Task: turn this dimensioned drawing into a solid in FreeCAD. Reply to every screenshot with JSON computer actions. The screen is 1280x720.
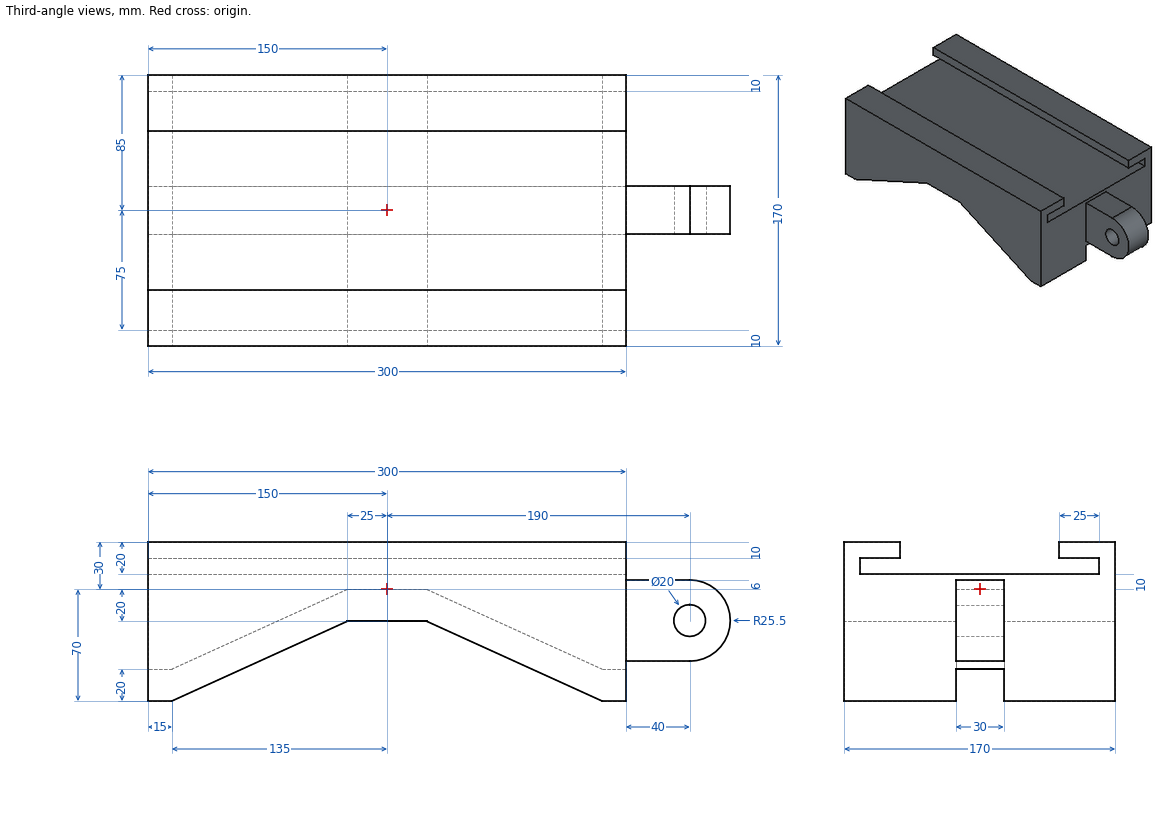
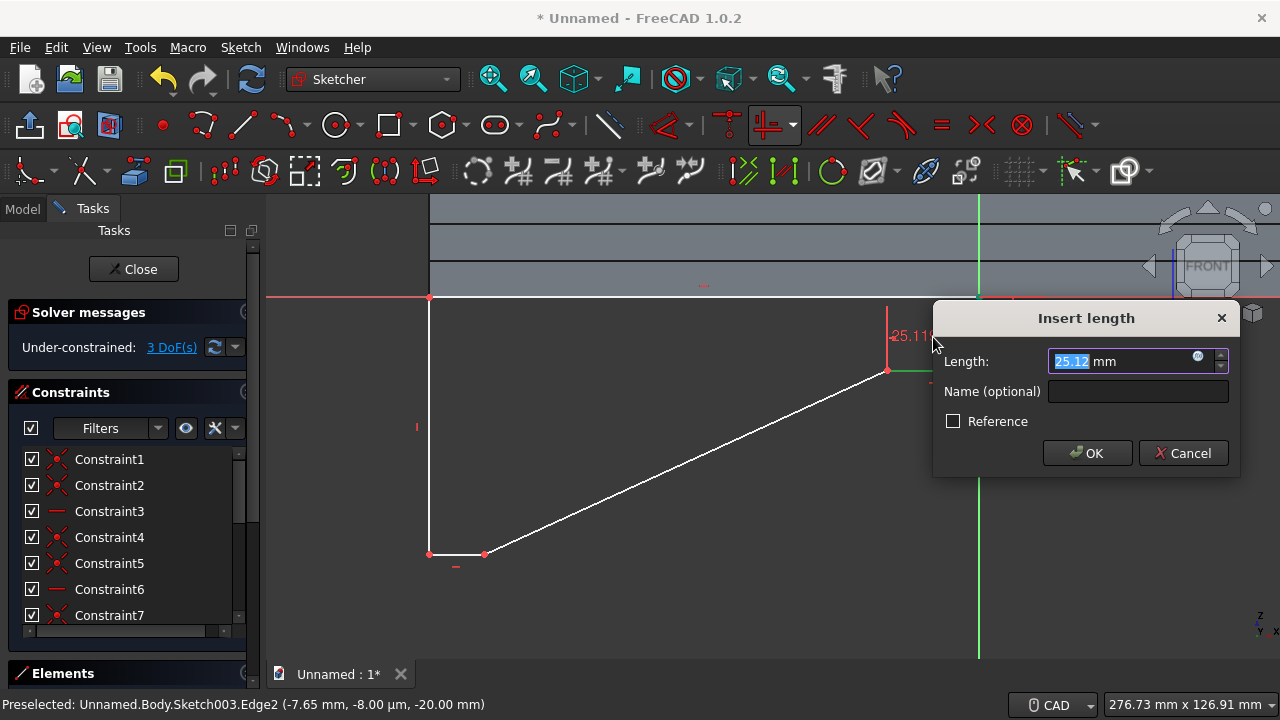
{"action": "type", "text": "25"}
{"action": "key", "text": "Return"}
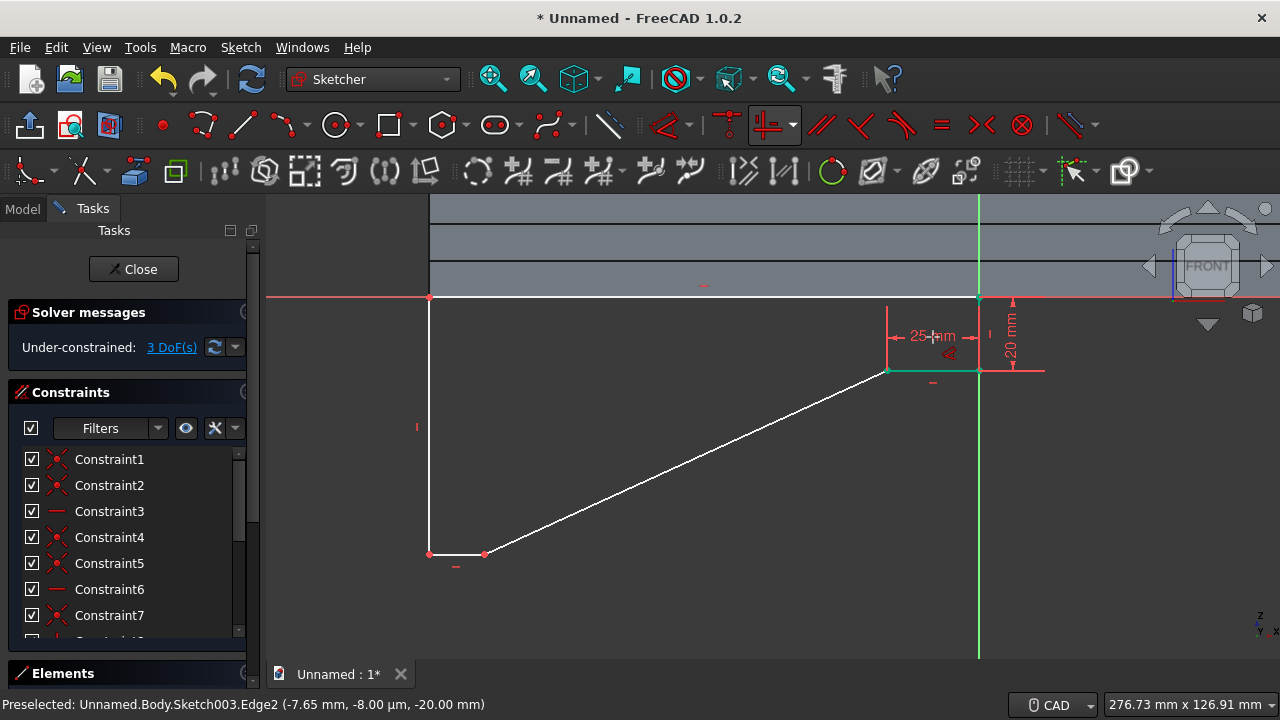
{"action": "left_click", "coordinate": [468, 555]}
{"action": "left_click", "coordinate": [457, 589]}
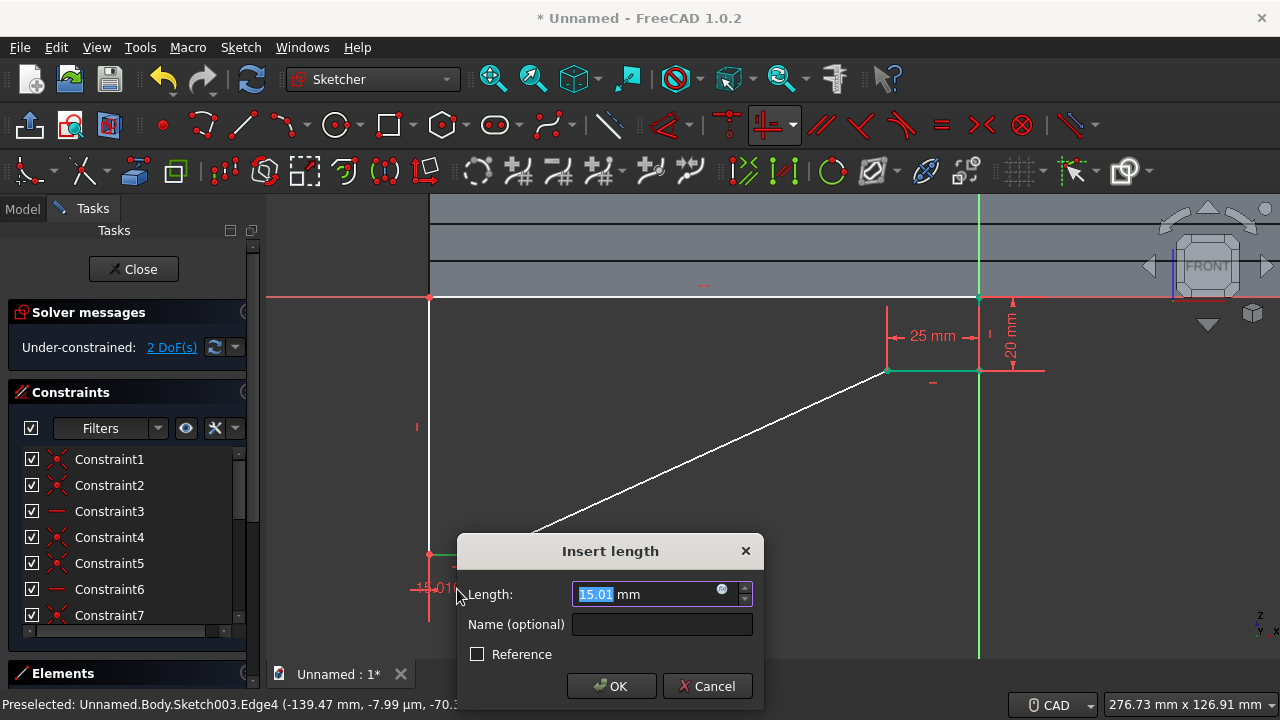
{"action": "type", "text": "15"}
{"action": "key", "text": "Return"}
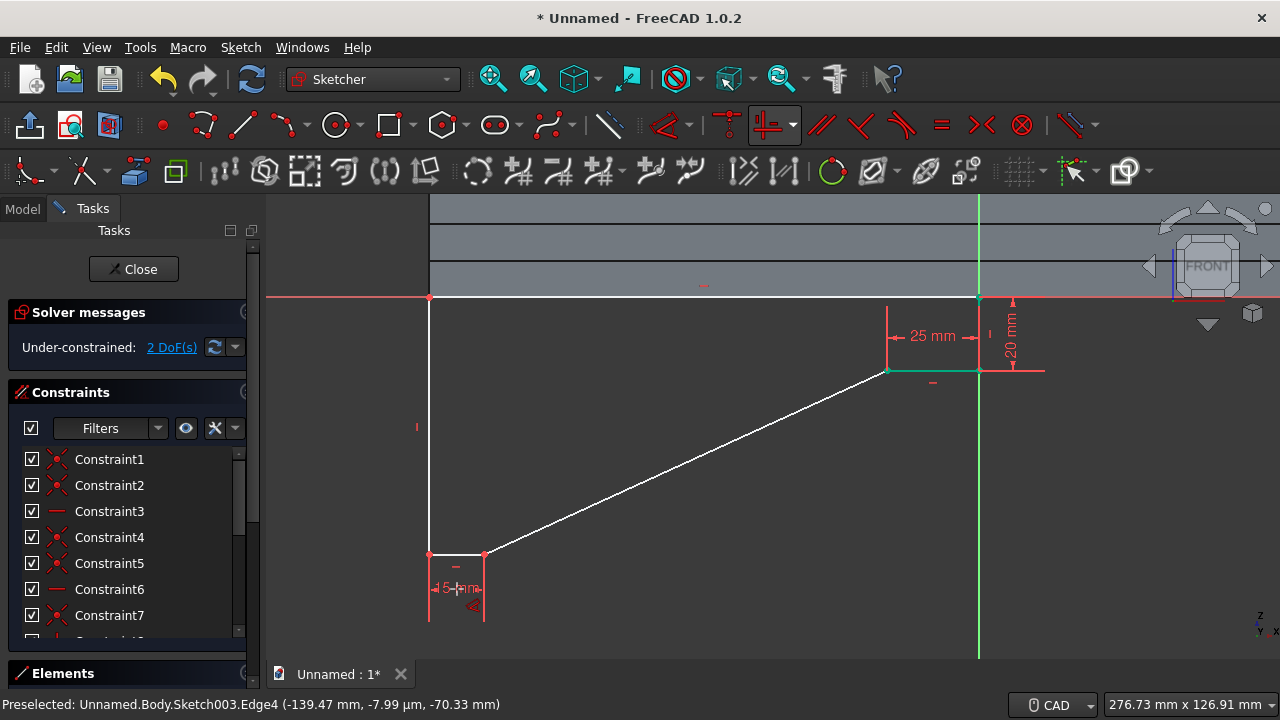
{"action": "left_click", "coordinate": [429, 478]}
{"action": "left_click", "coordinate": [395, 426]}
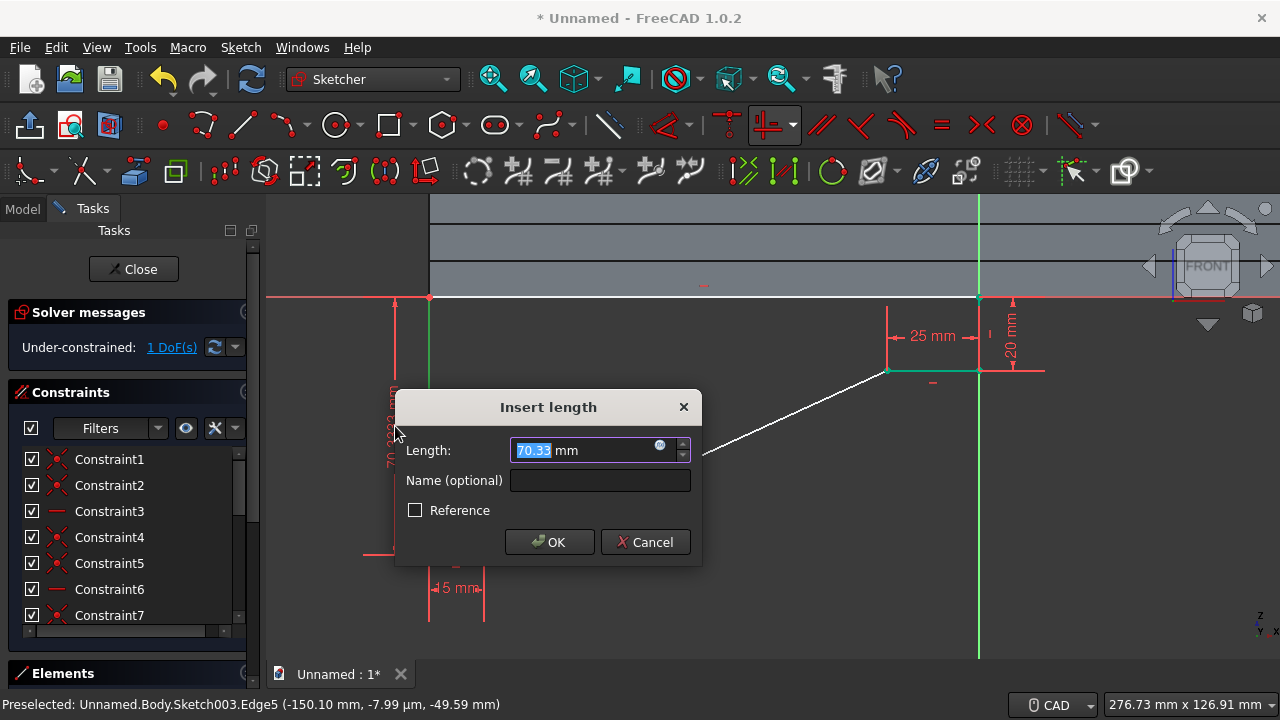
{"action": "type", "text": "70"}
{"action": "key", "text": "Return"}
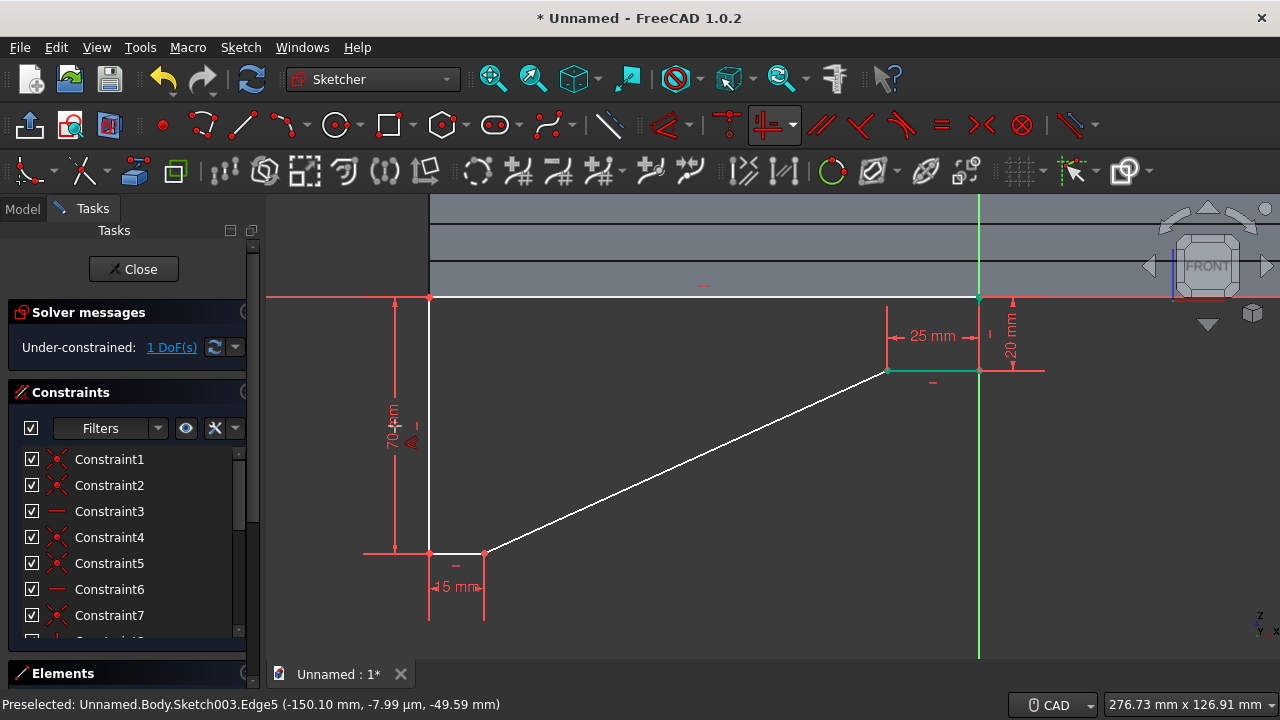
{"action": "left_click", "coordinate": [594, 297]}
{"action": "left_click", "coordinate": [704, 263]}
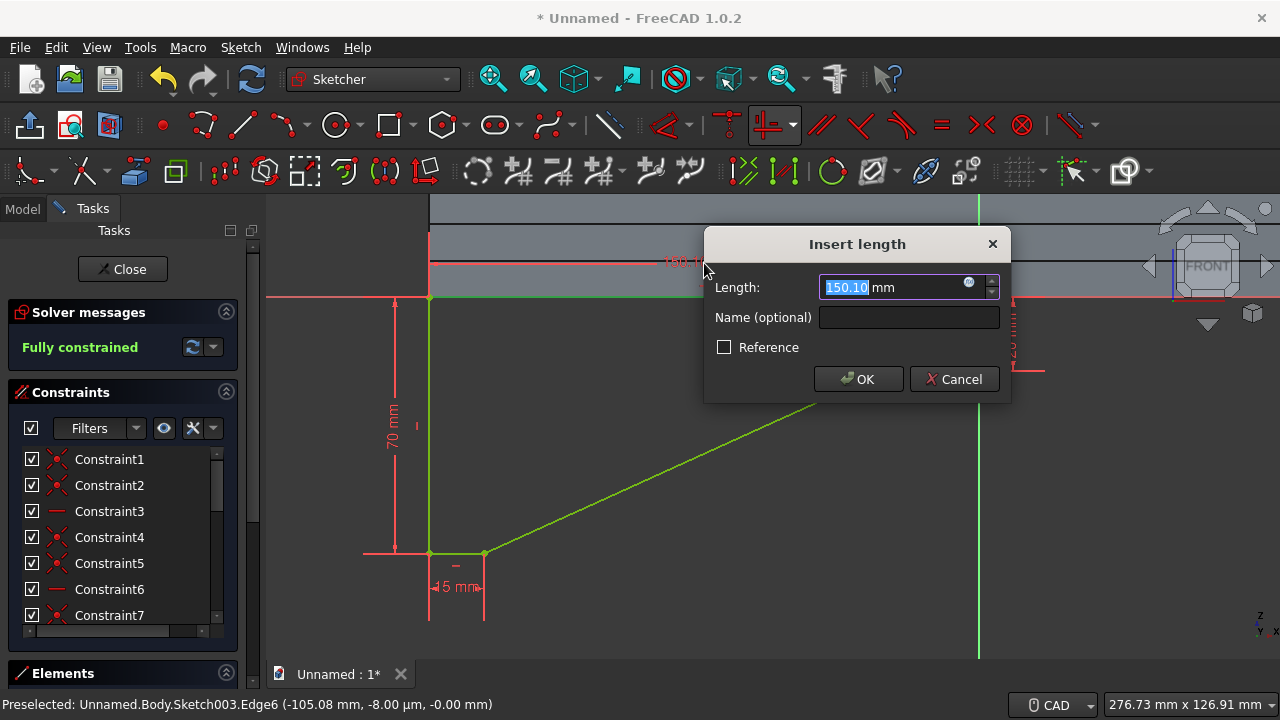
{"action": "type", "text": "150"}
{"action": "key", "text": "Return"}
{"action": "key", "text": "Escape"}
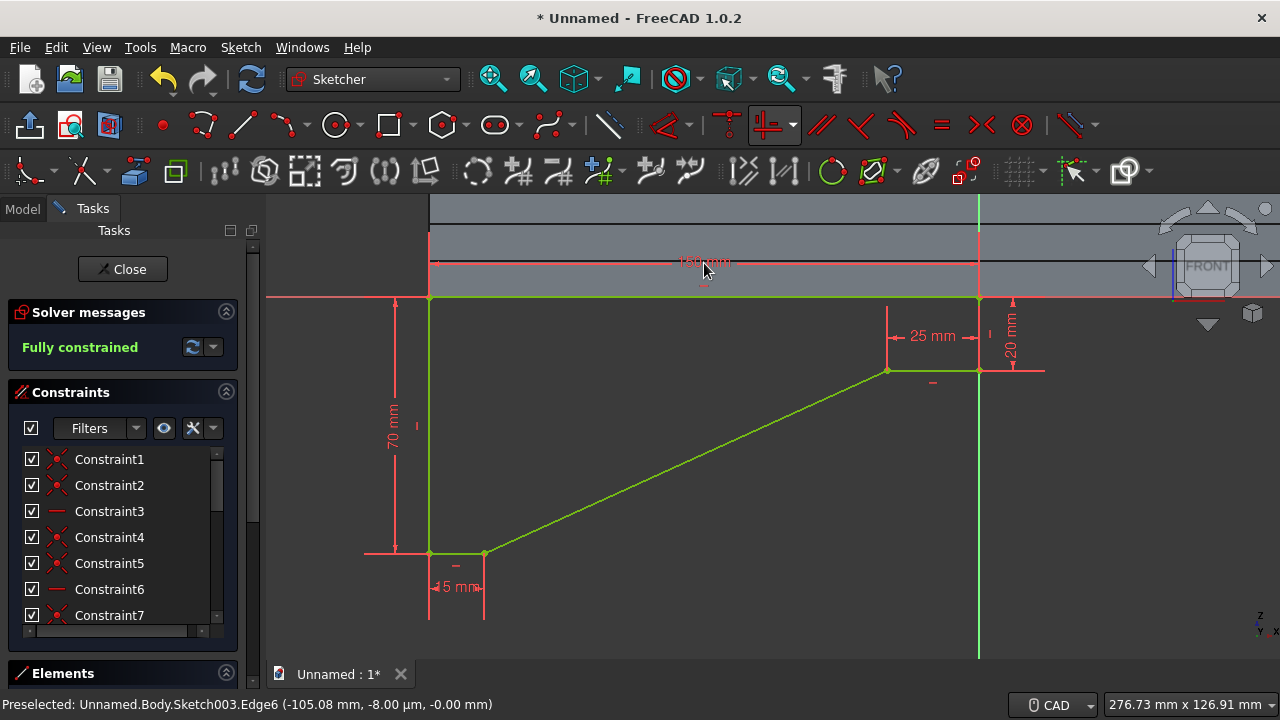
{"action": "left_click", "coordinate": [123, 269]}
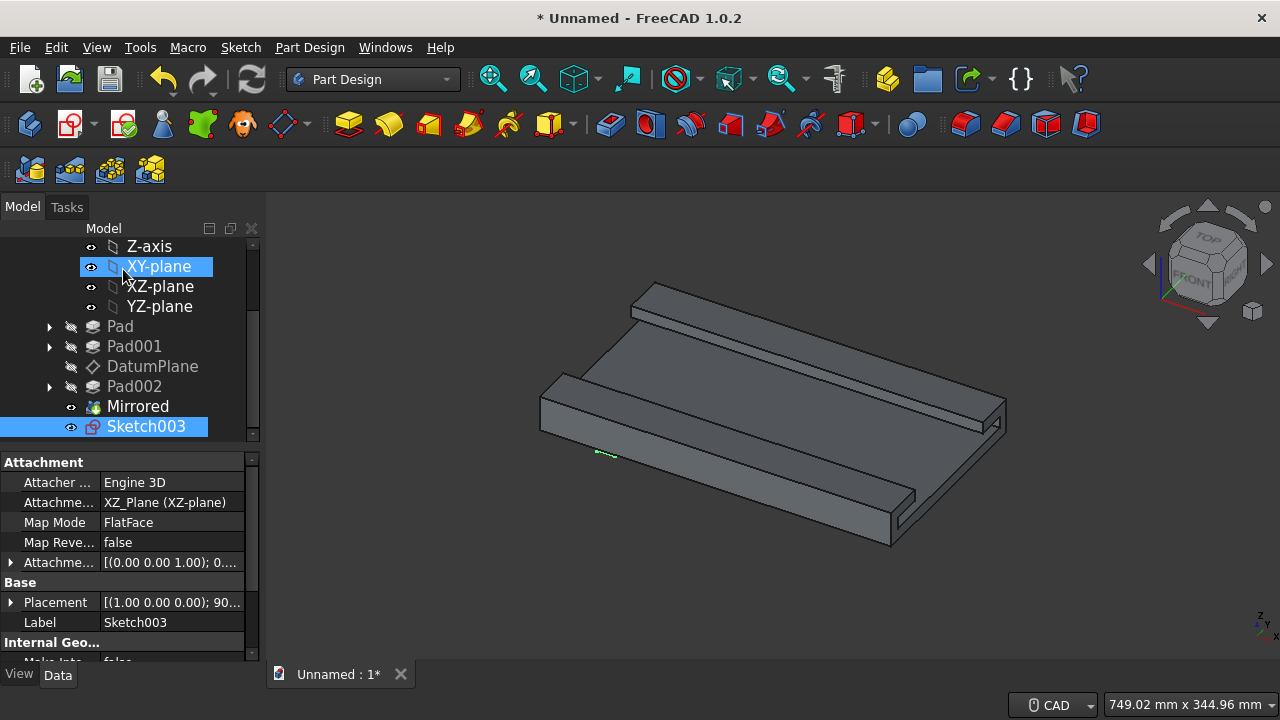
{"action": "left_click", "coordinate": [350, 124]}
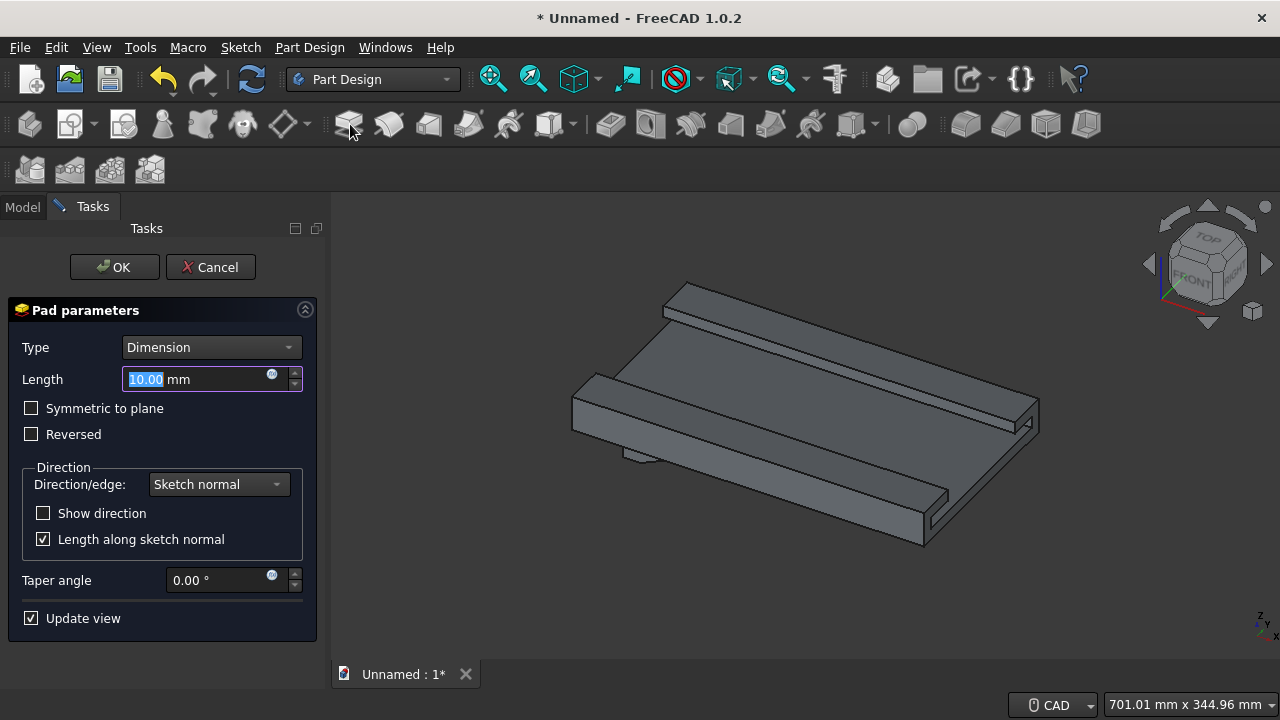
{"action": "type", "text": "170"}
{"action": "key", "text": "Tab"}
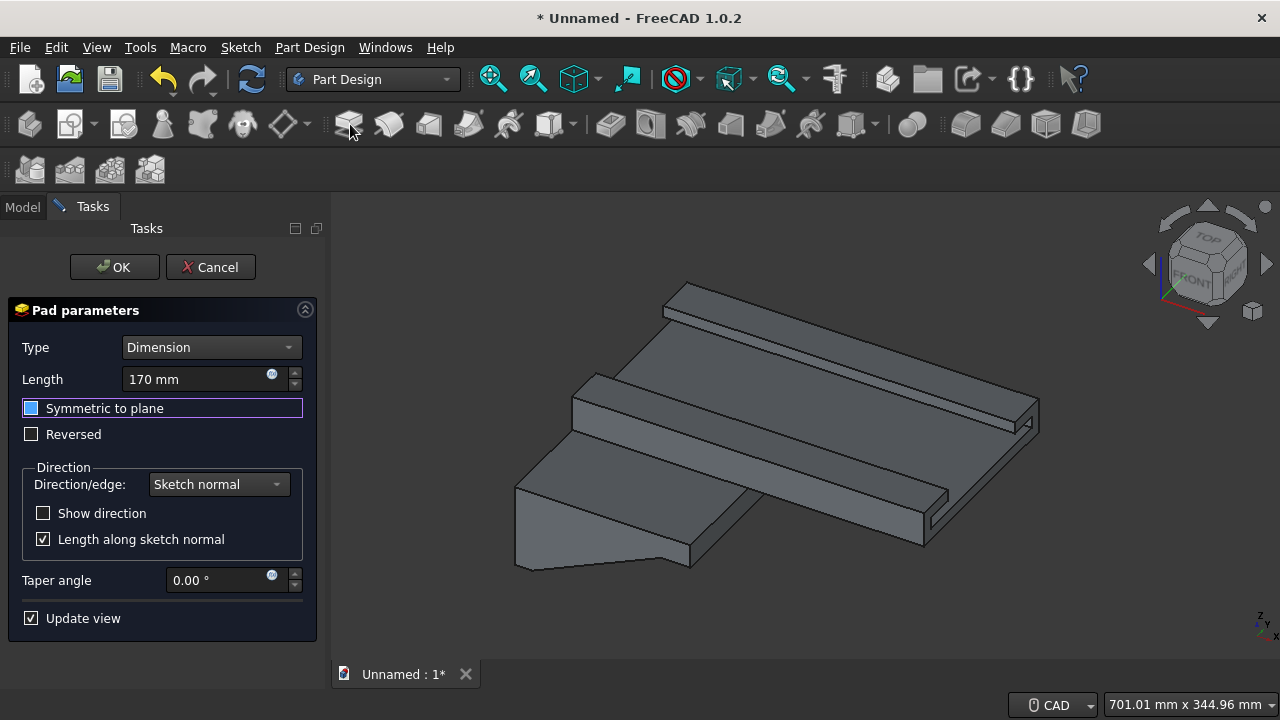
{"action": "left_click", "coordinate": [30, 408]}